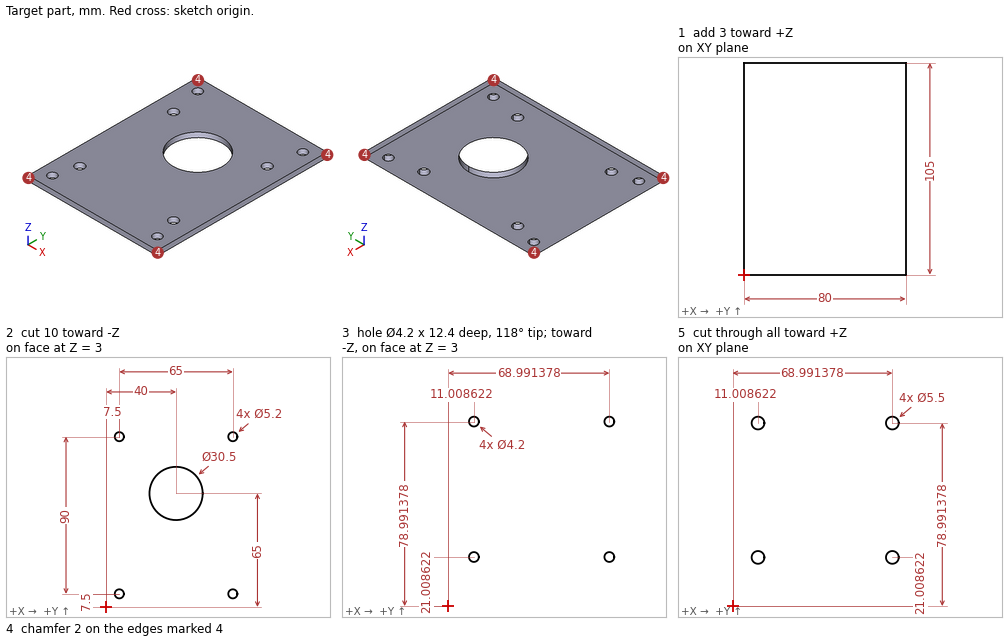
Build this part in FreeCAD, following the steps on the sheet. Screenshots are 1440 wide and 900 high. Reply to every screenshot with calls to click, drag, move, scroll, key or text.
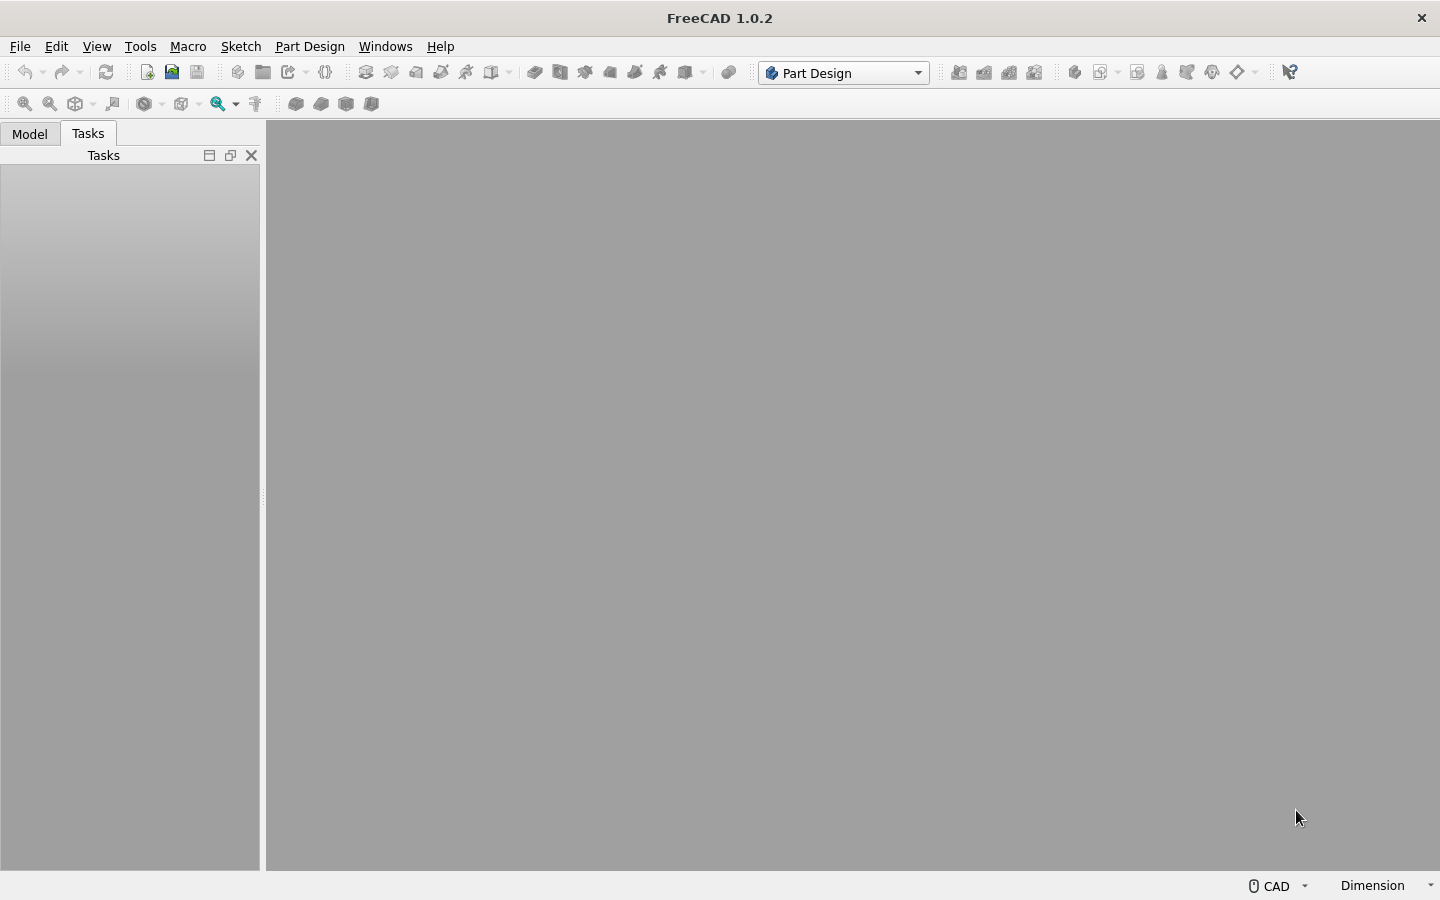
click(147, 72)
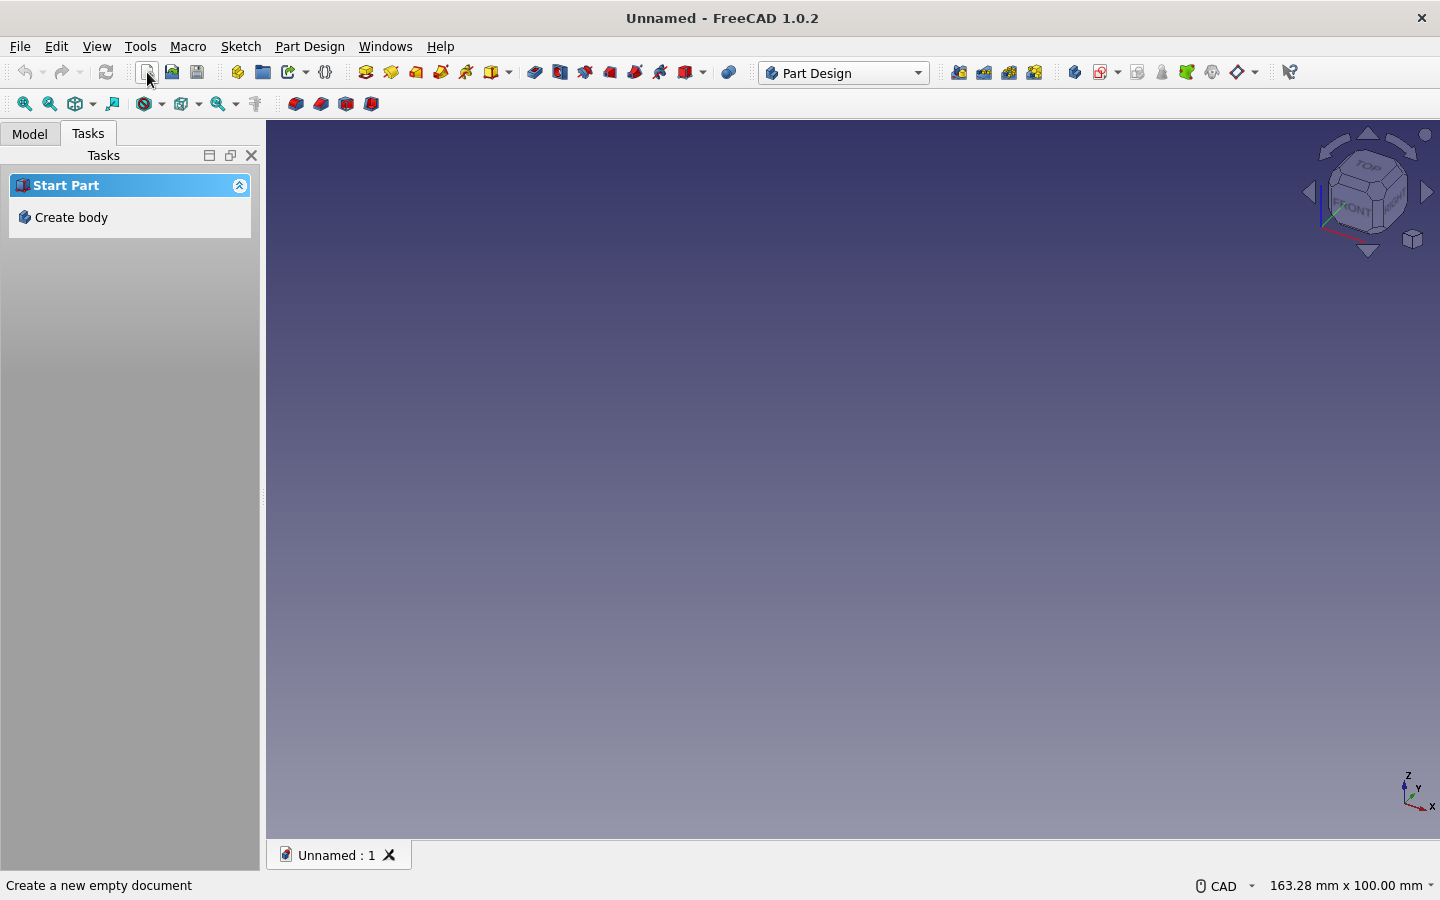
click(1100, 72)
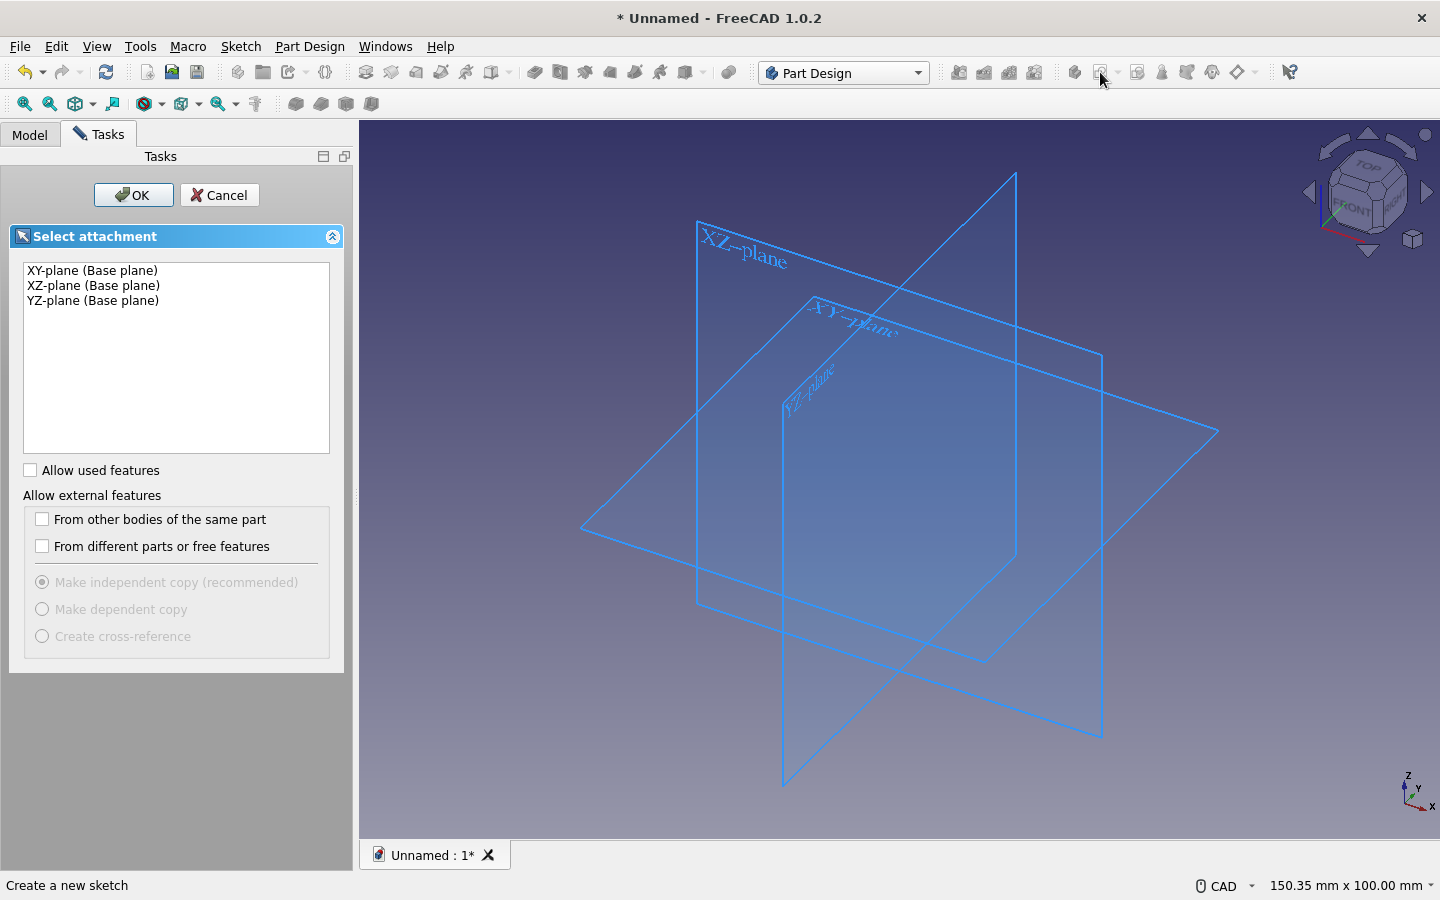
click(84, 270)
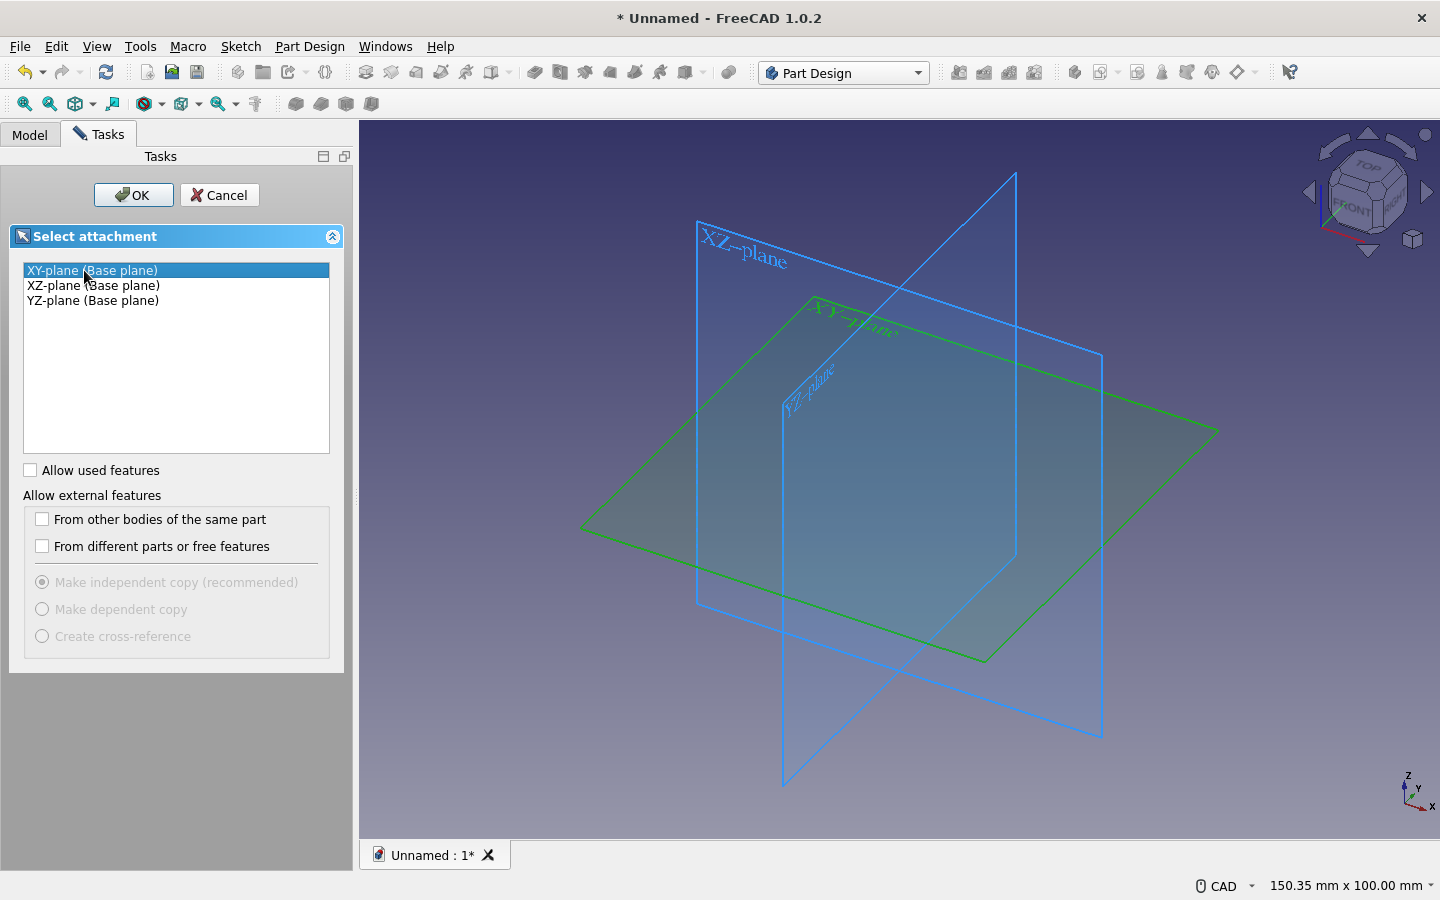
click(134, 195)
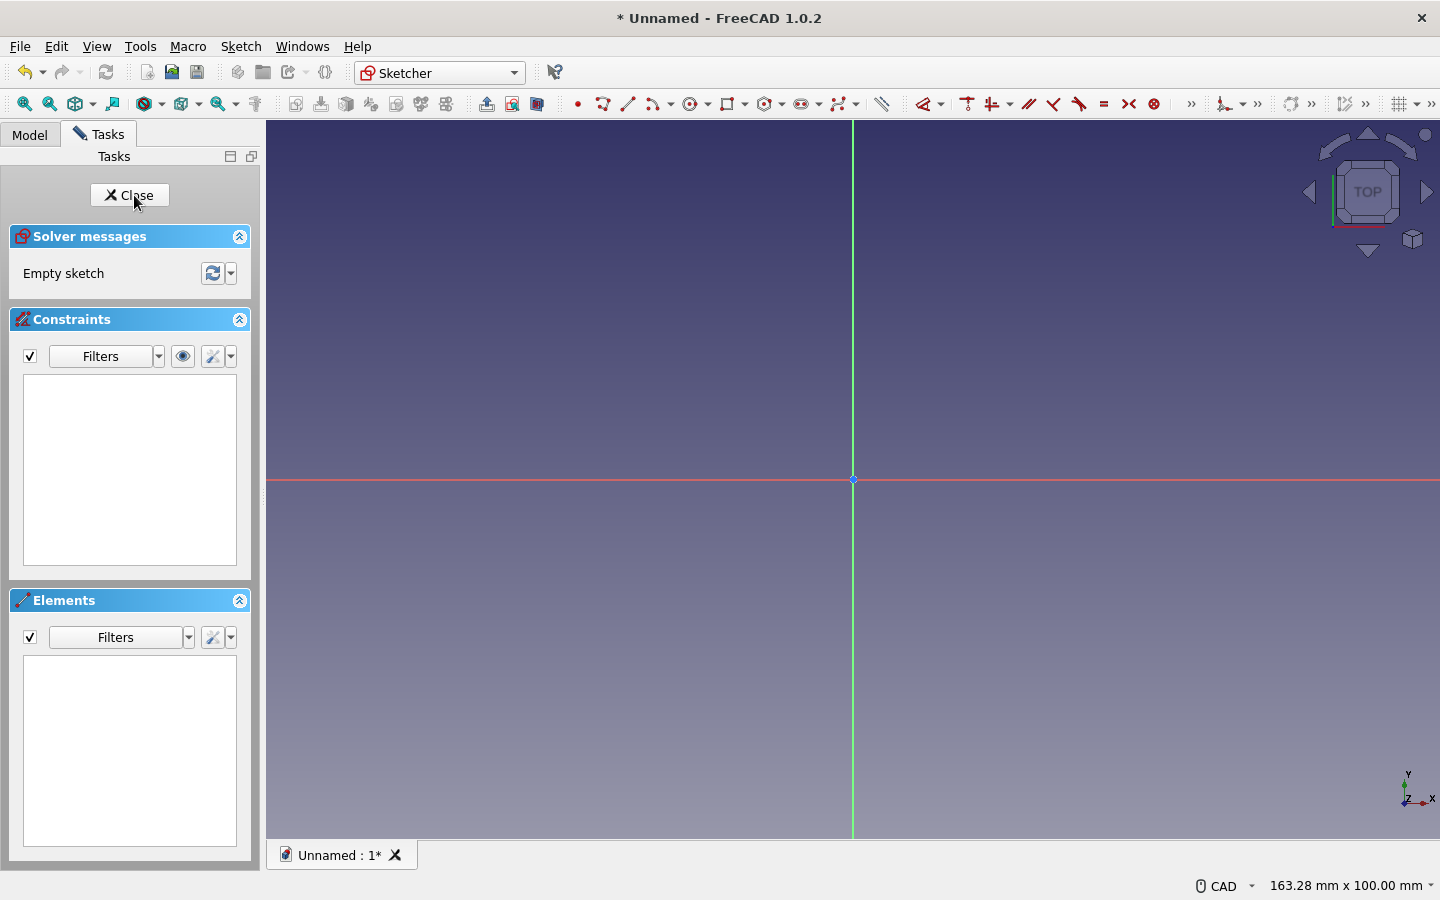
scroll(351, 811, down, 3)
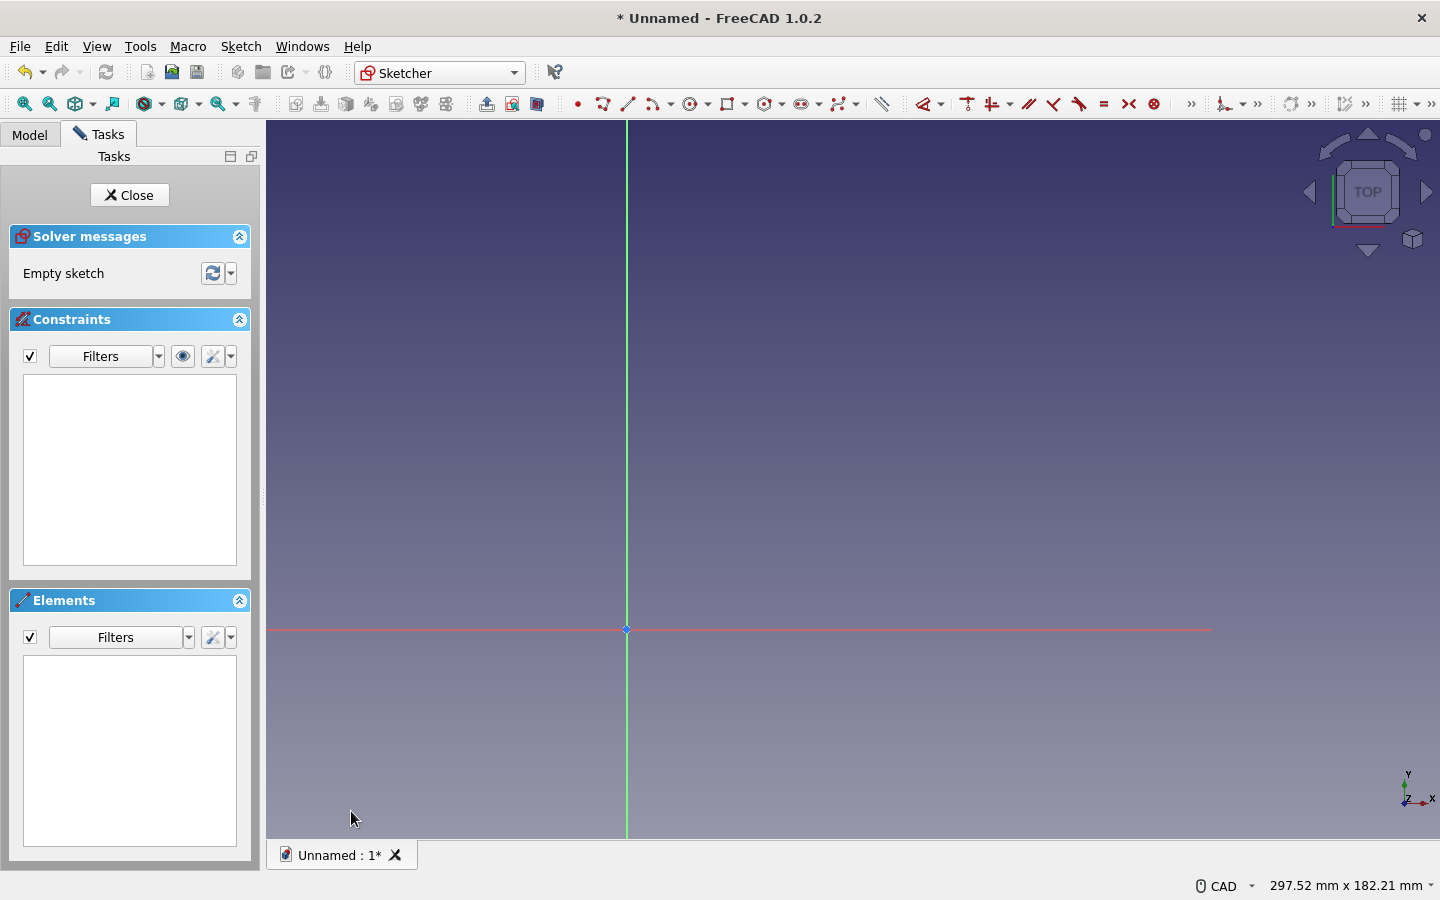
click(726, 104)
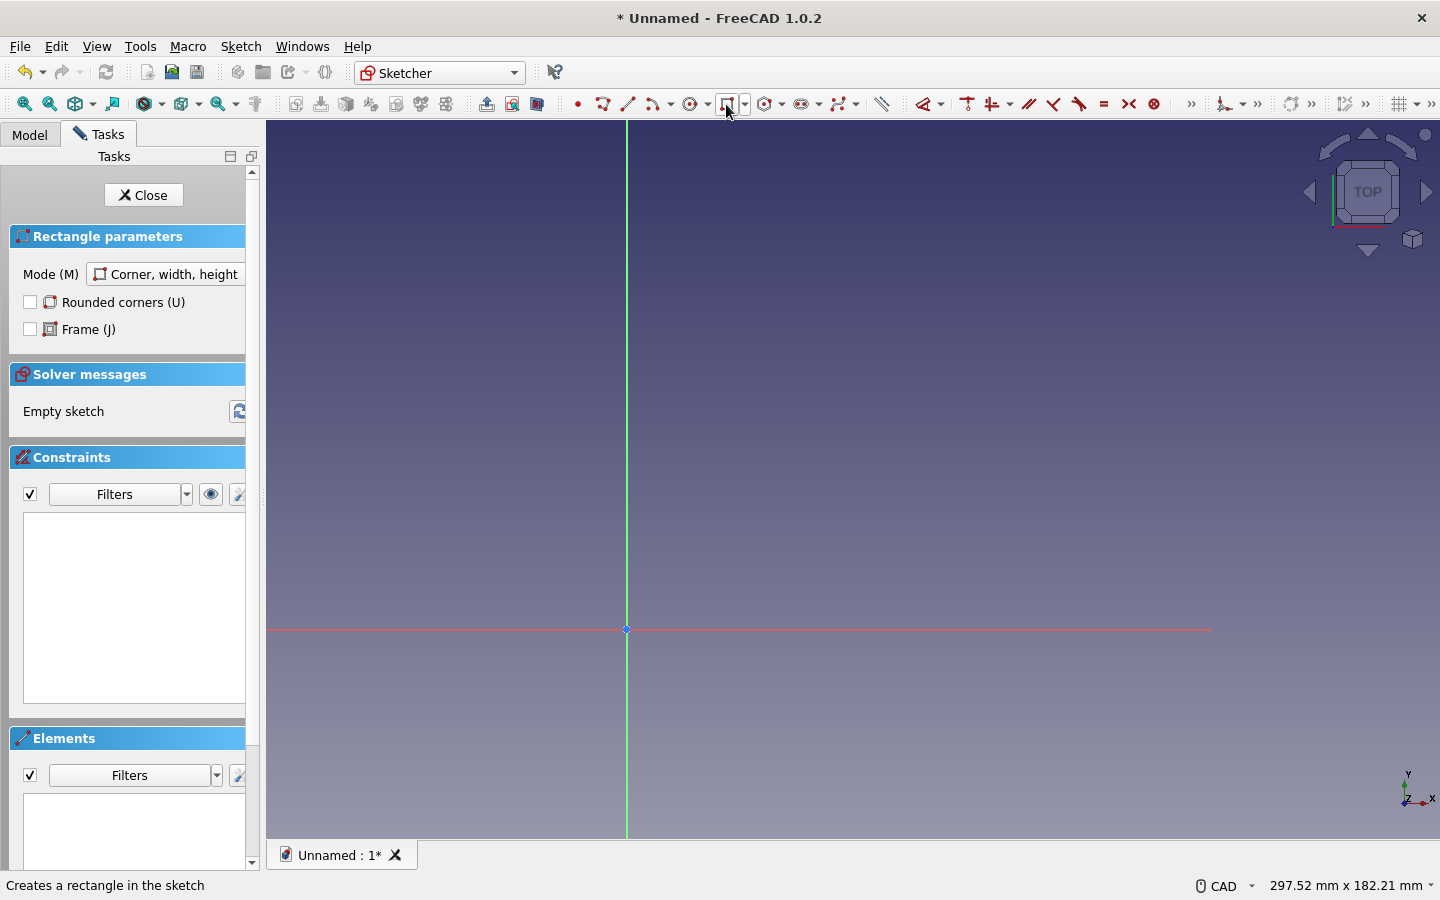
click(627, 630)
click(942, 215)
key(Escape)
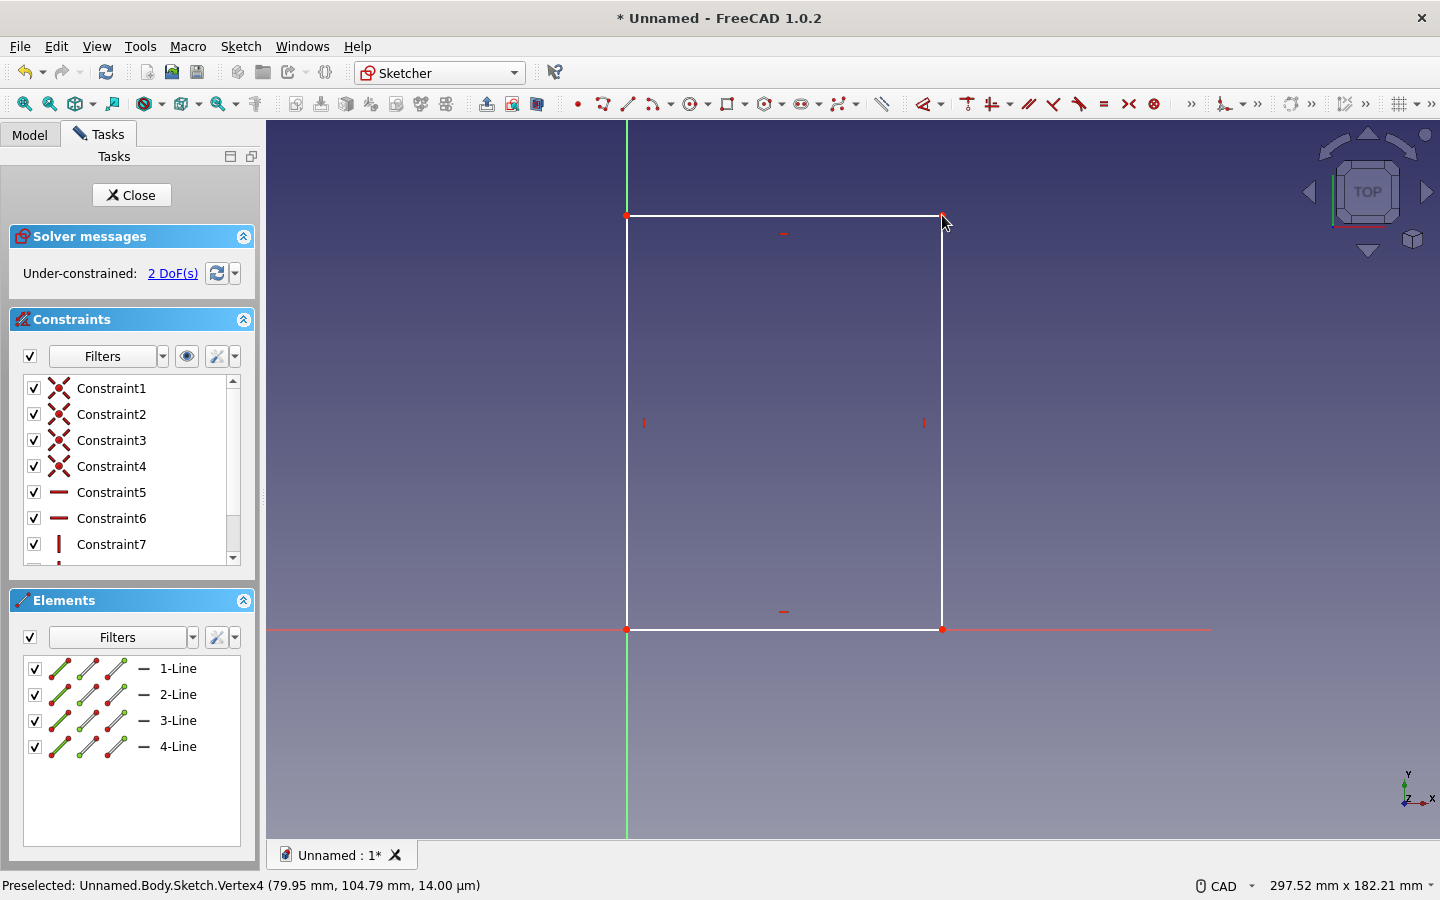
click(922, 104)